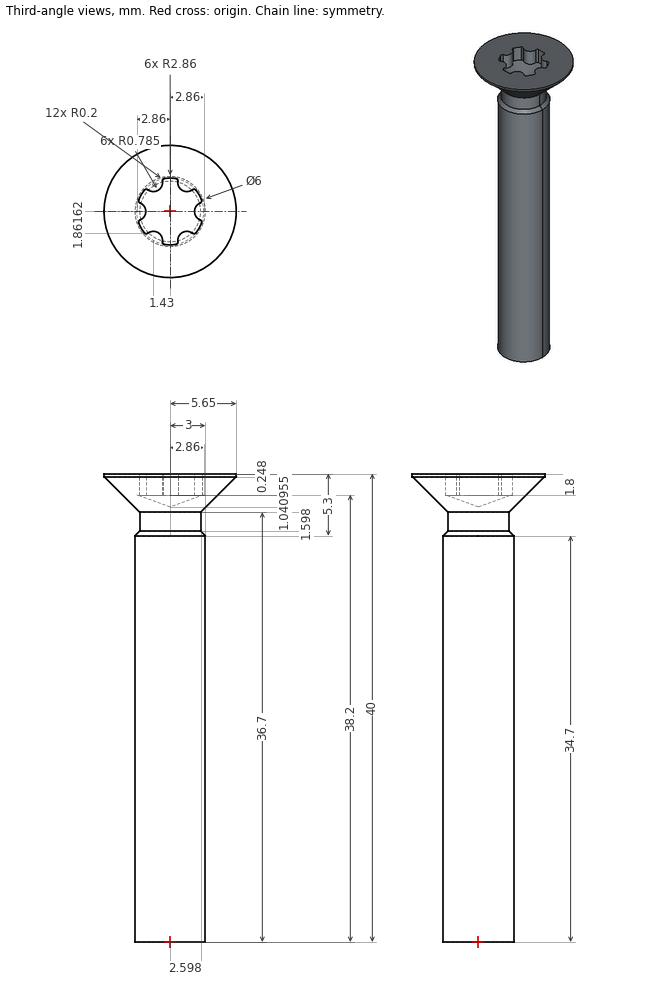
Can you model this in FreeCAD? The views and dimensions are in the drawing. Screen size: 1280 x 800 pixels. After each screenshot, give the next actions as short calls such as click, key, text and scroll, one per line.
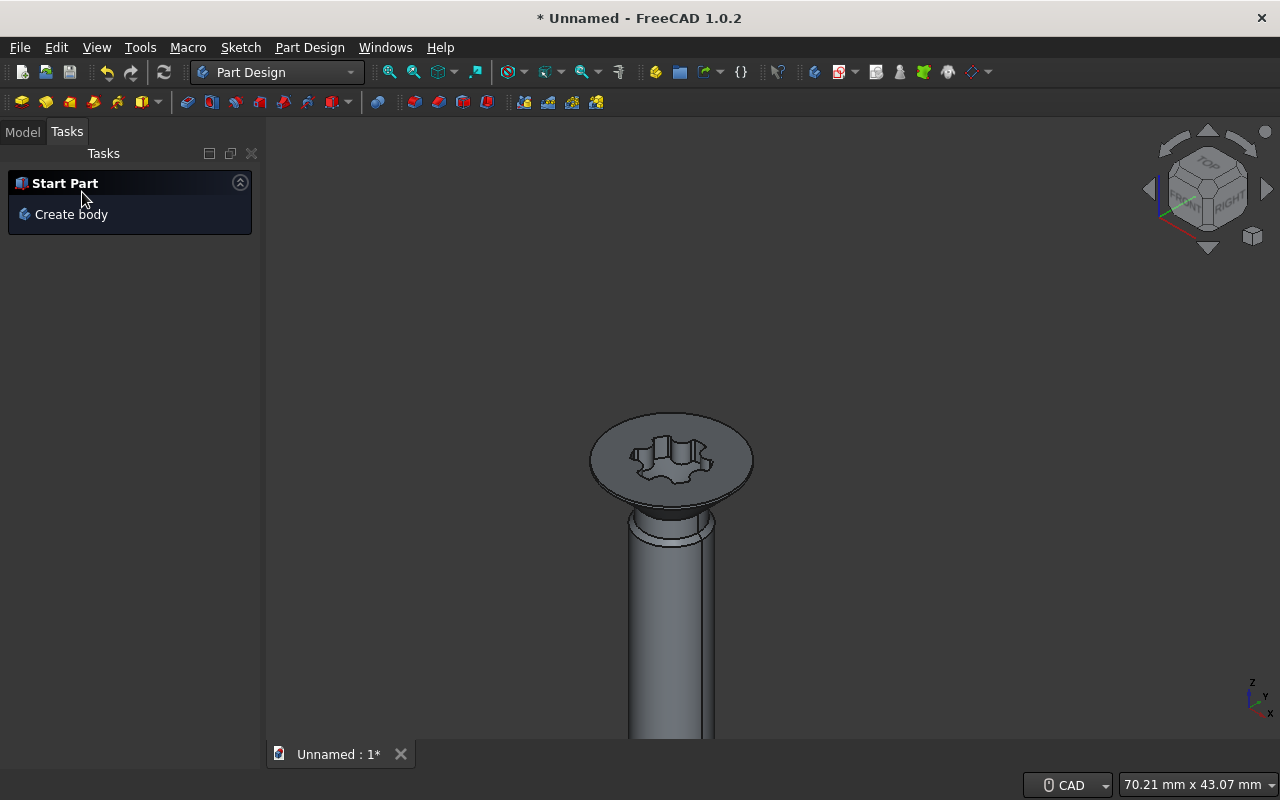
click(390, 72)